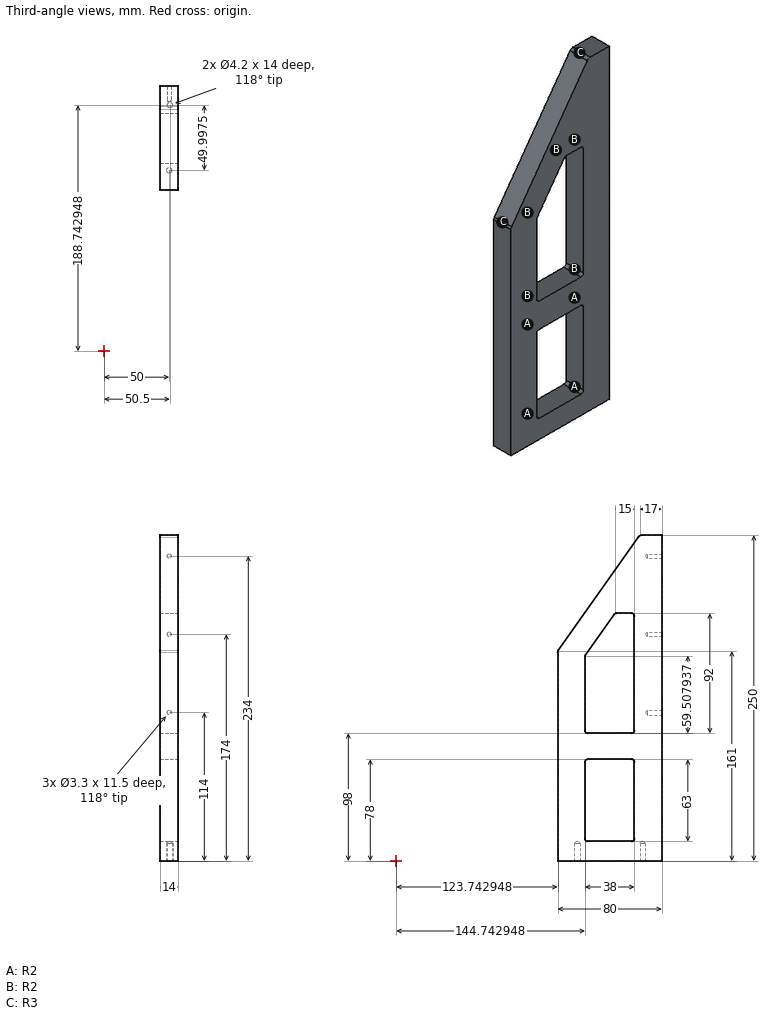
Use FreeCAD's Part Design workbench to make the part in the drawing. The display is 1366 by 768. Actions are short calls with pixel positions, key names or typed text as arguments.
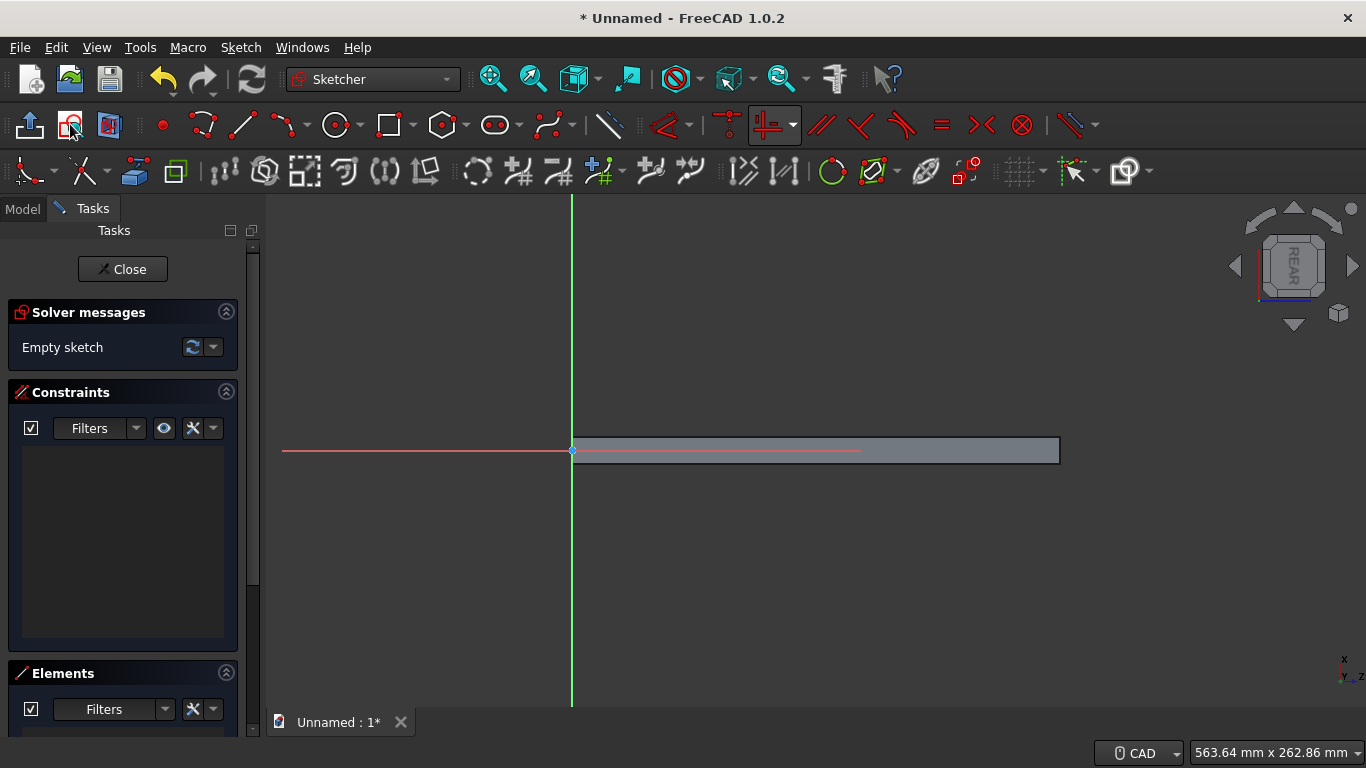
scroll(913, 451, up, 2)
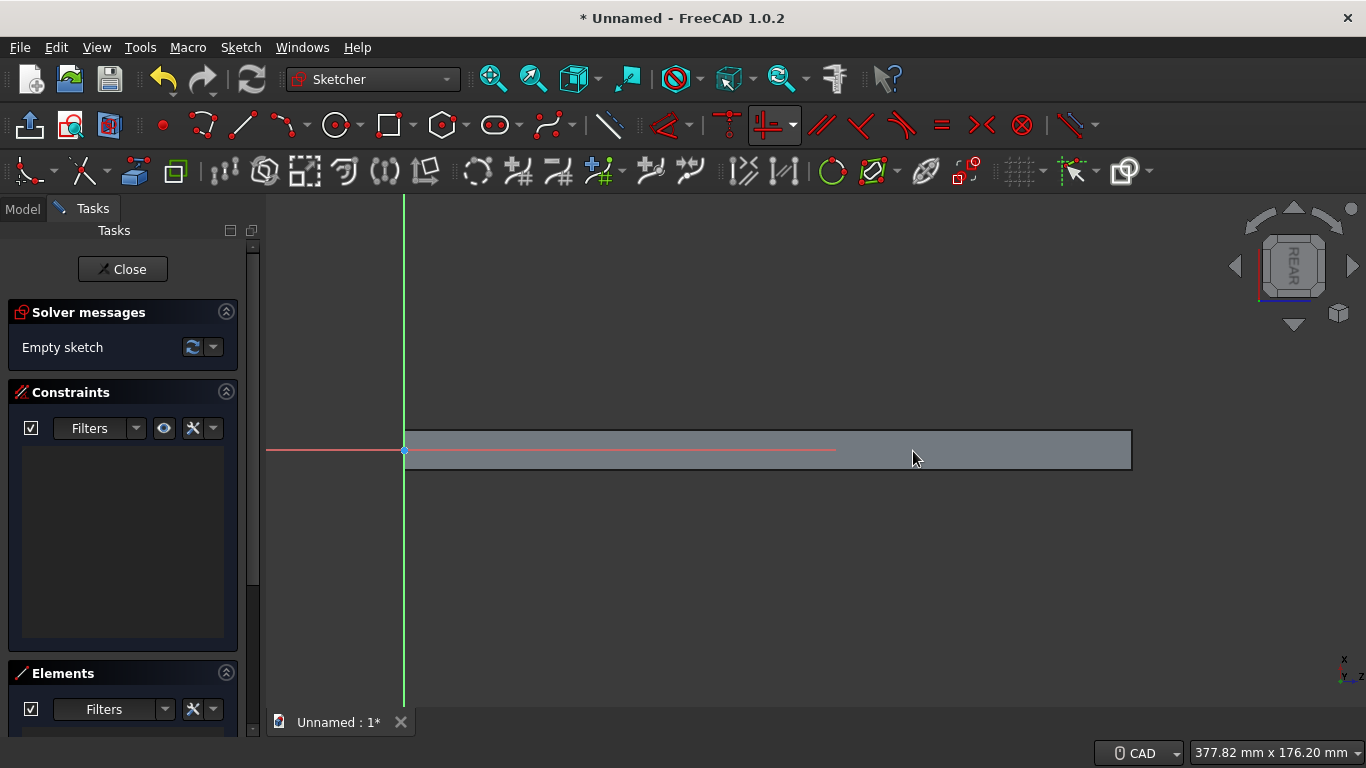
click(336, 126)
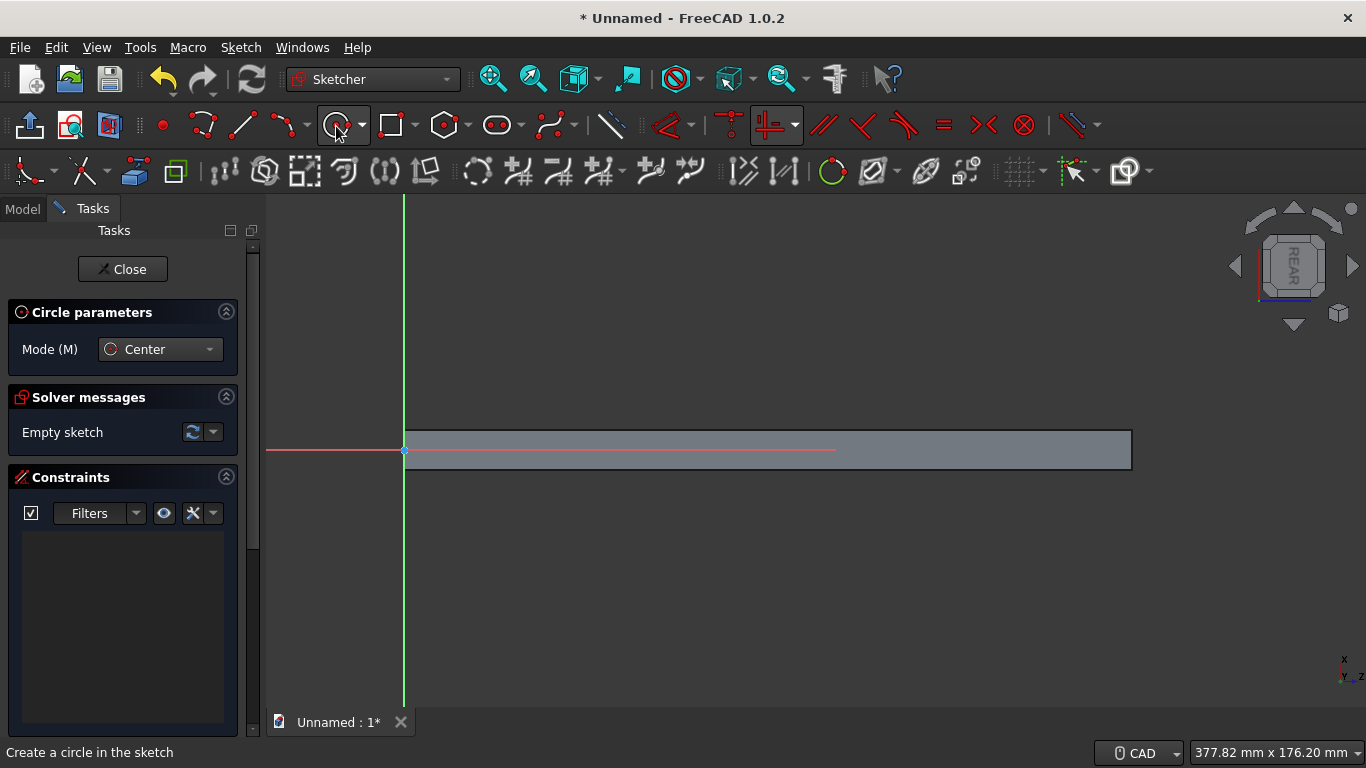
scroll(736, 450, up, 8)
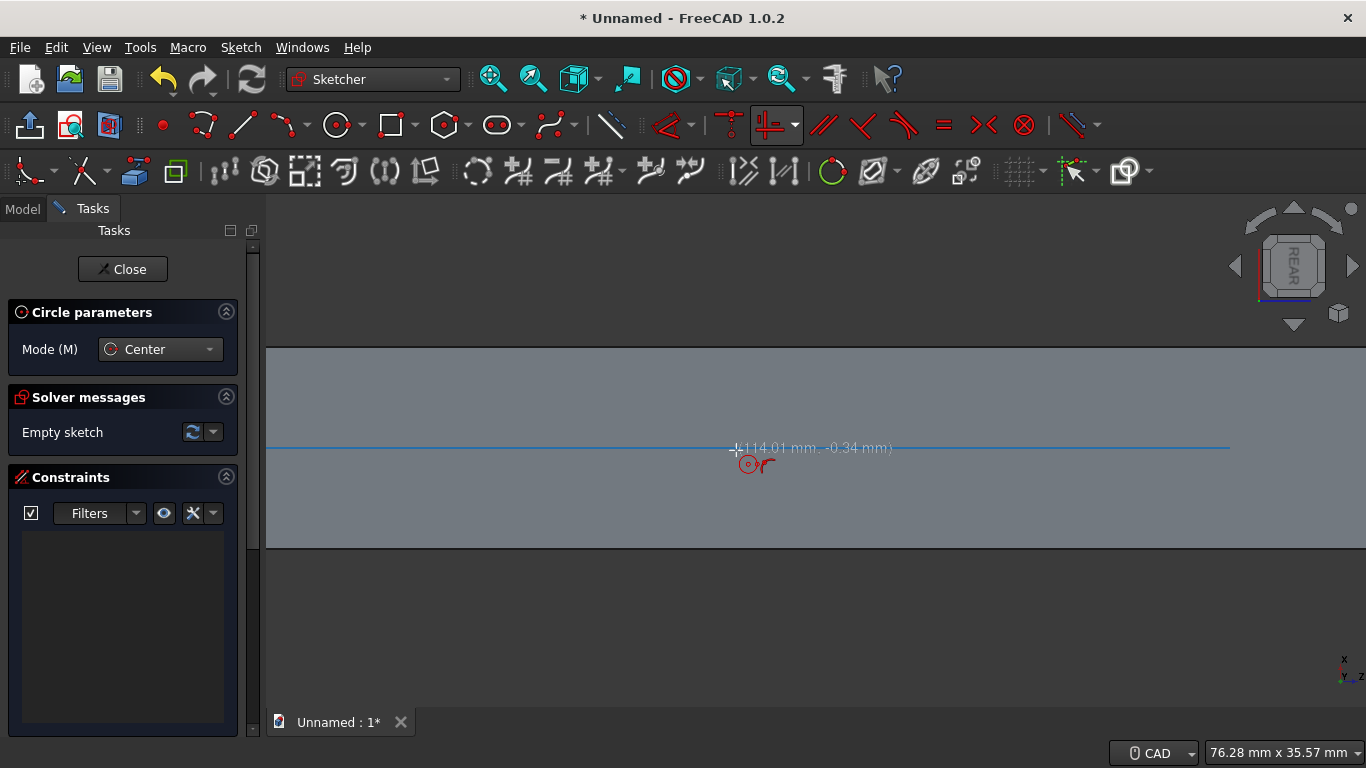
scroll(737, 451, down, 8)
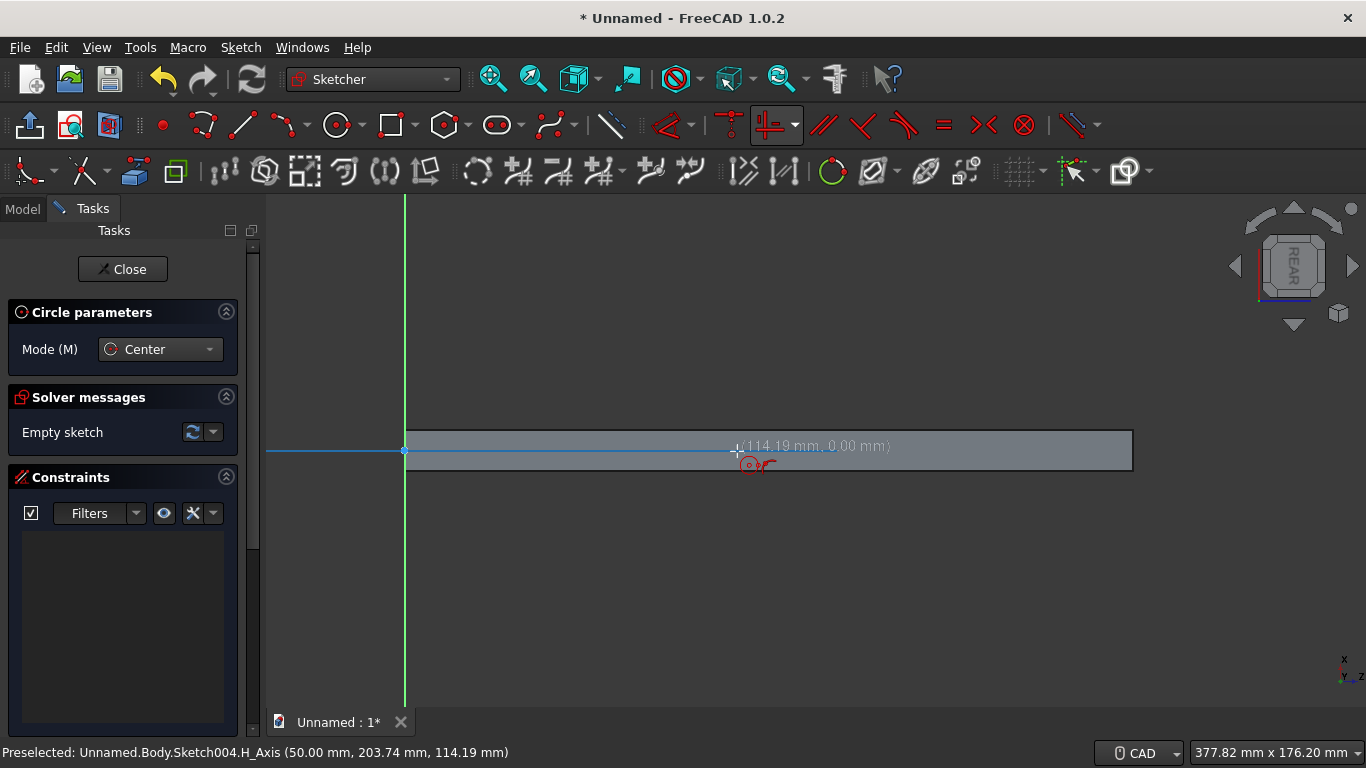
click(737, 451)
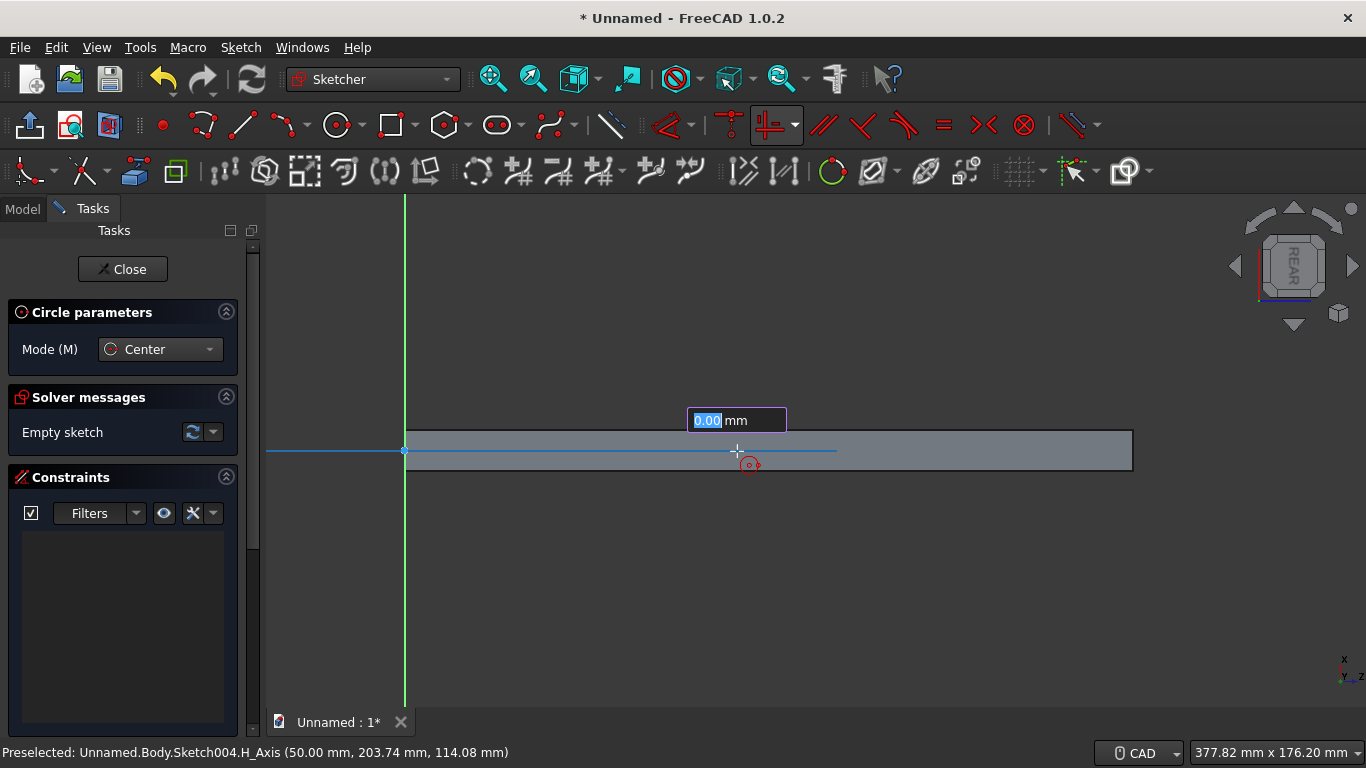
scroll(735, 455, up, 7)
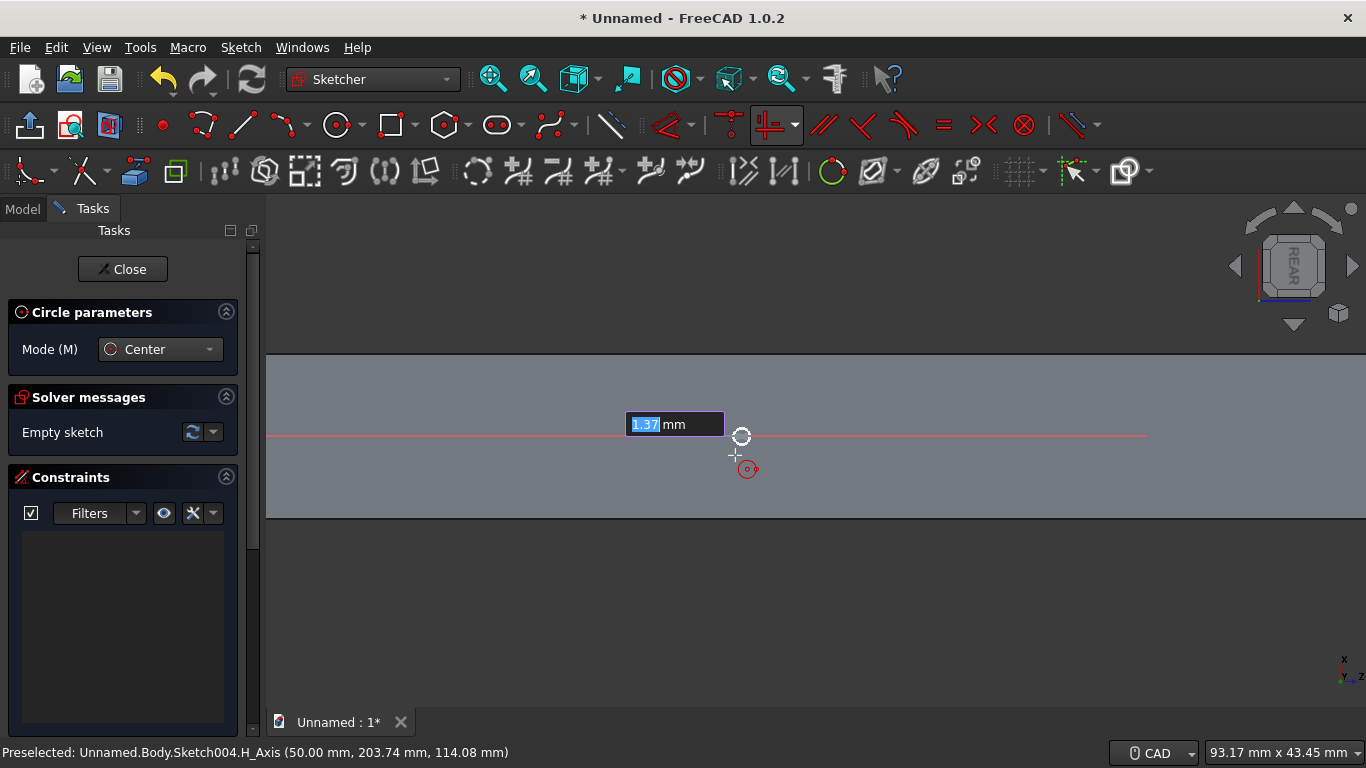
click(734, 455)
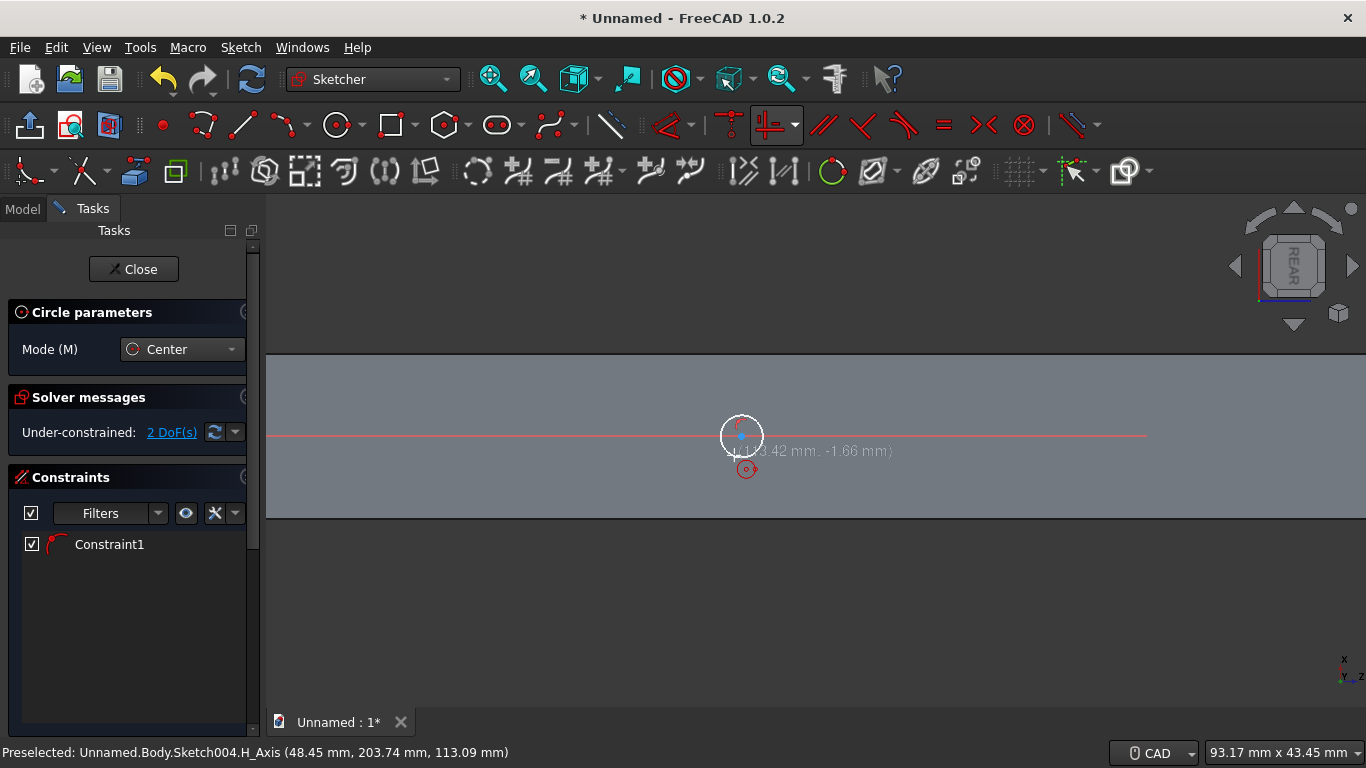
scroll(735, 455, down, 7)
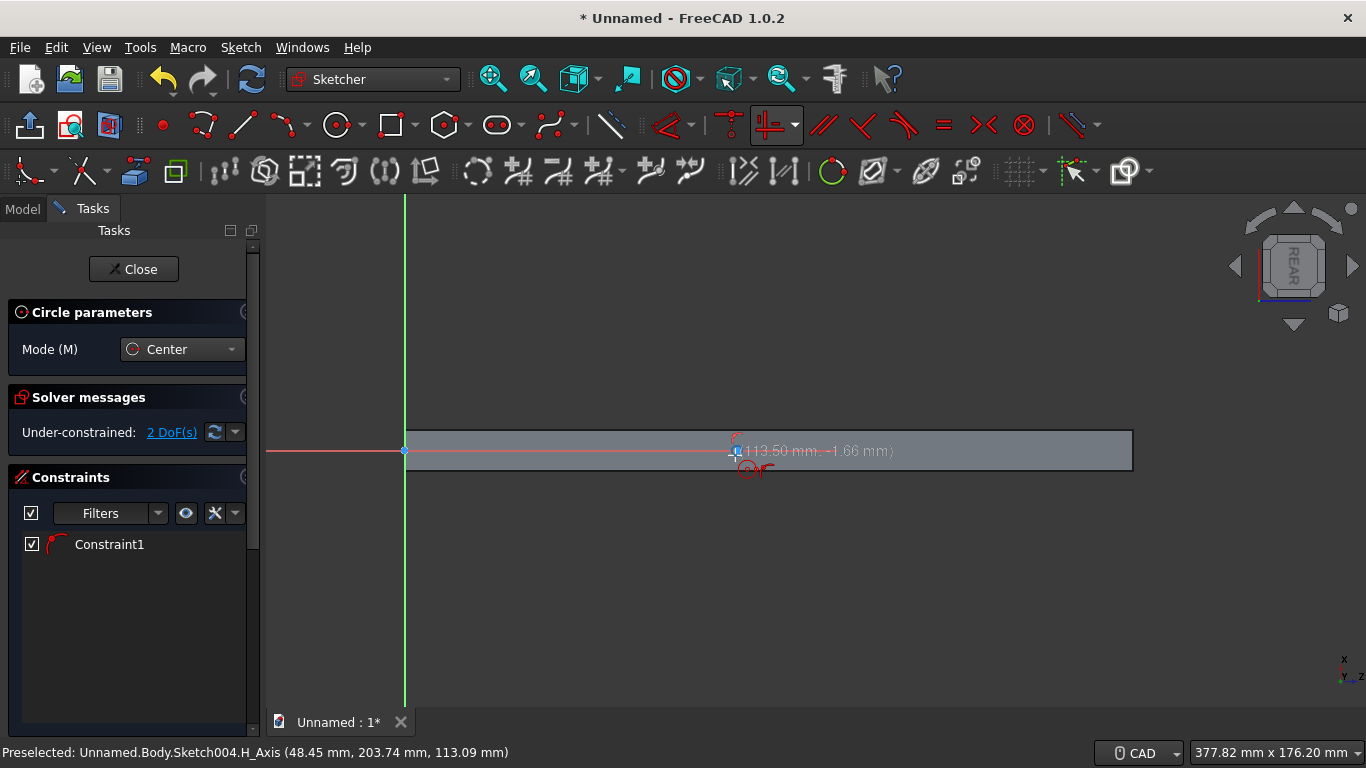
scroll(911, 451, up, 8)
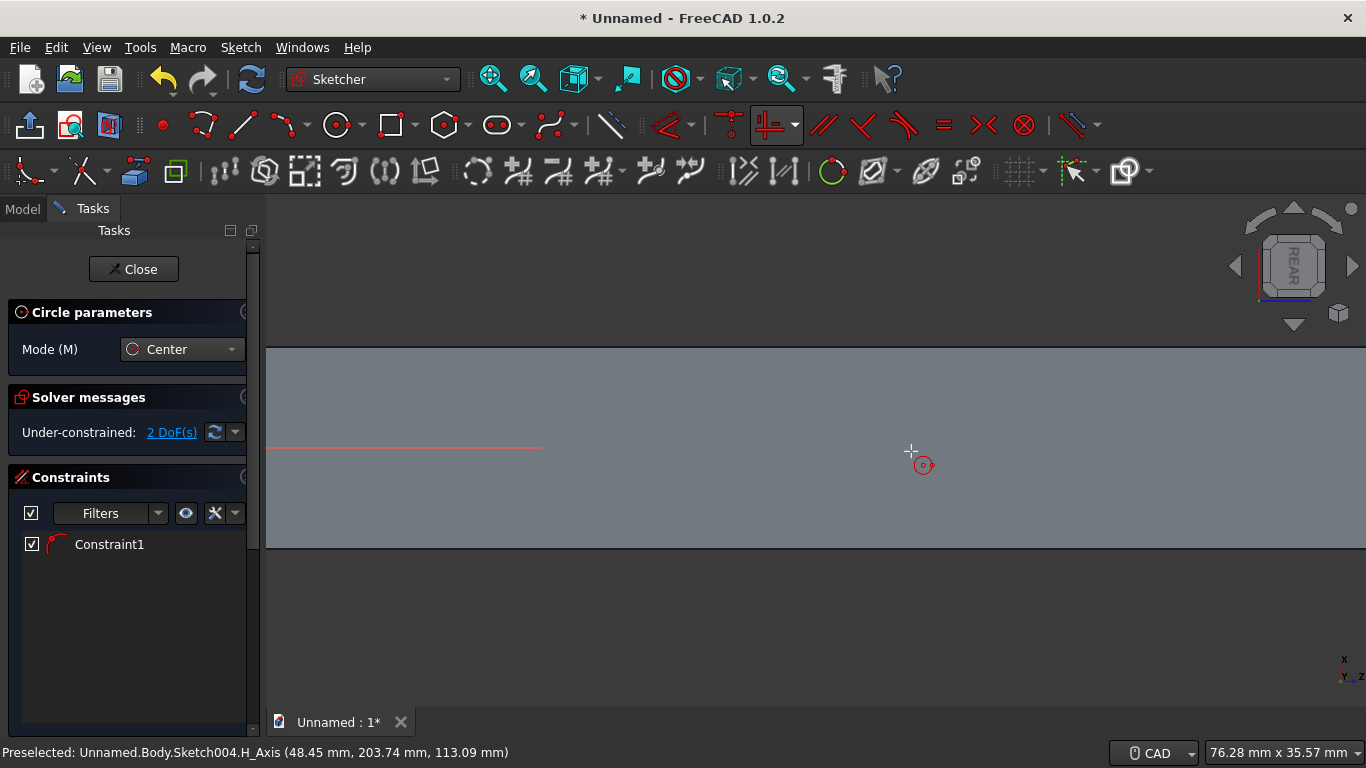
scroll(911, 451, down, 8)